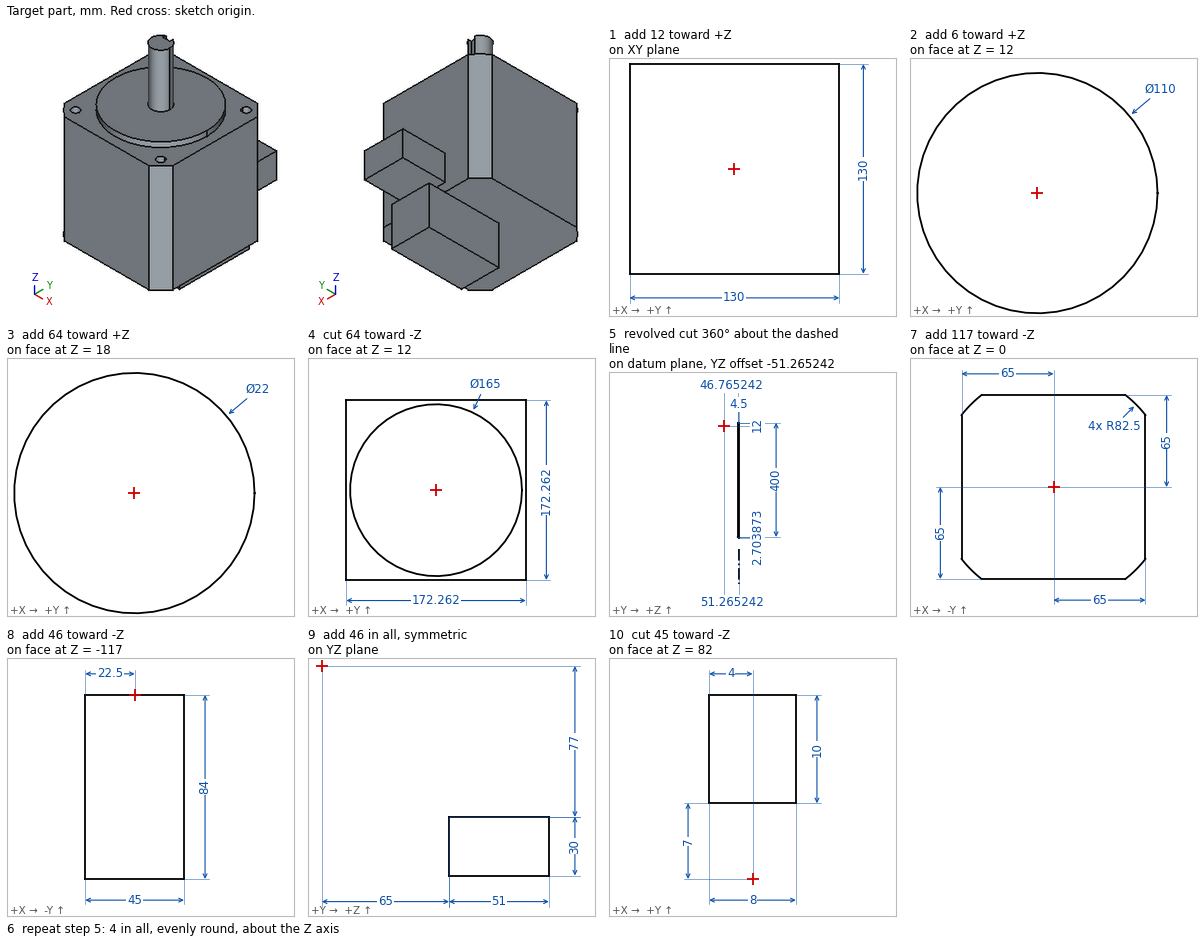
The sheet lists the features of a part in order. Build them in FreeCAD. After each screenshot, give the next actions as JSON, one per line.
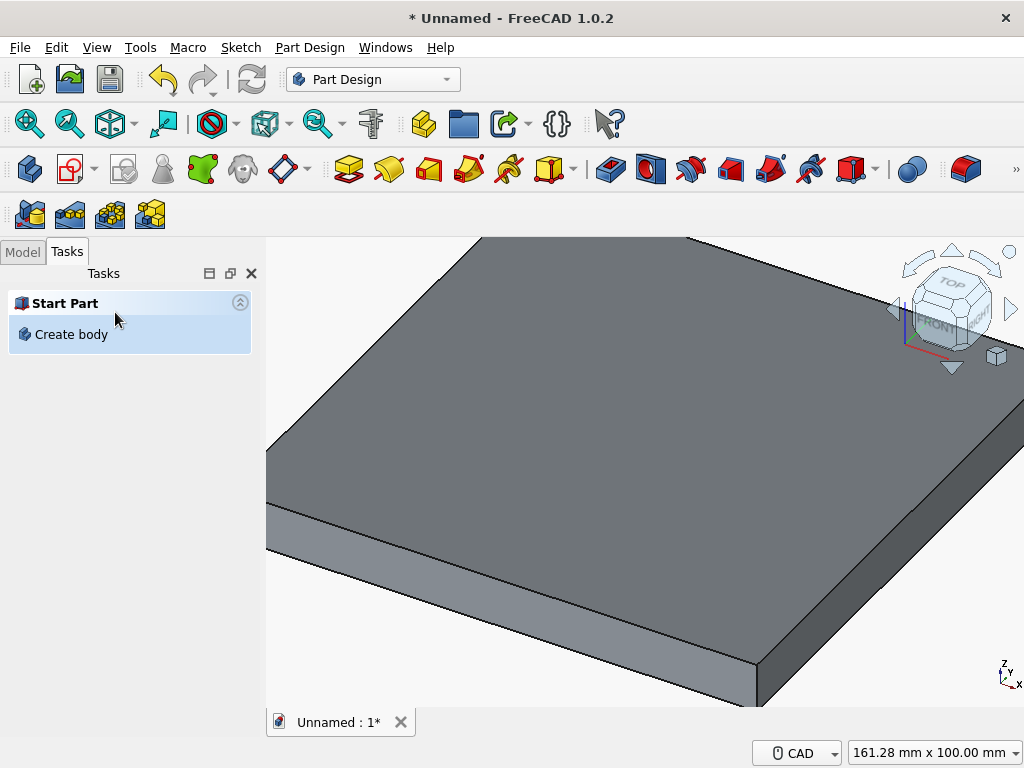
{"action": "left_click", "coordinate": [30, 124]}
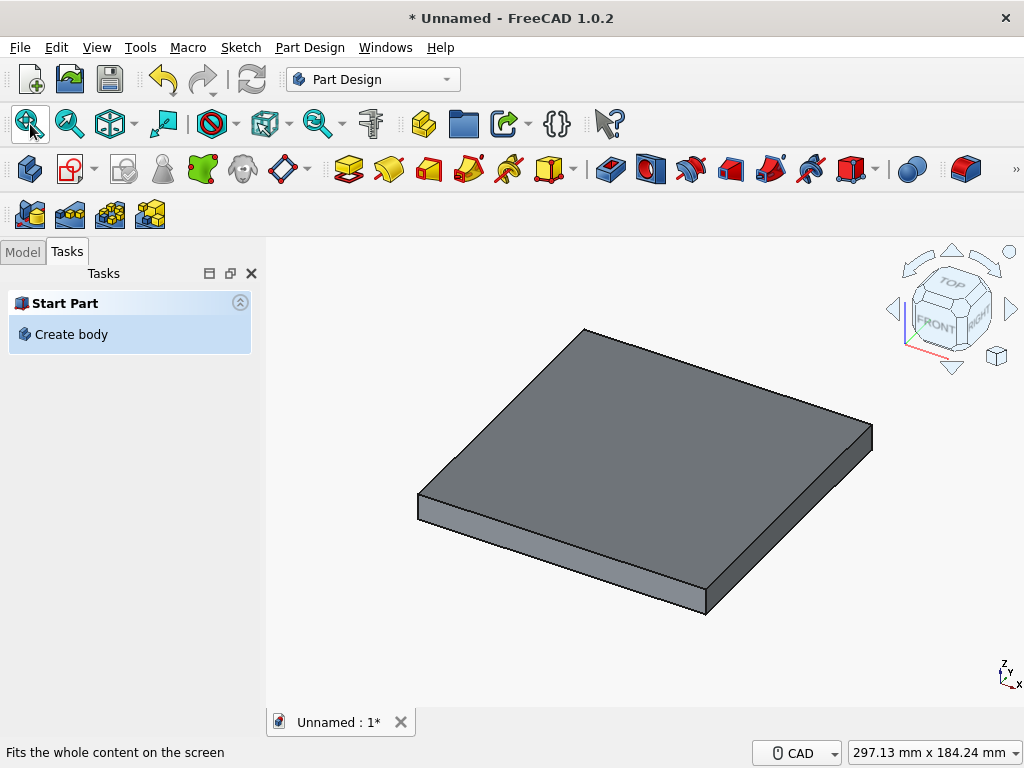
{"action": "left_click", "coordinate": [645, 458]}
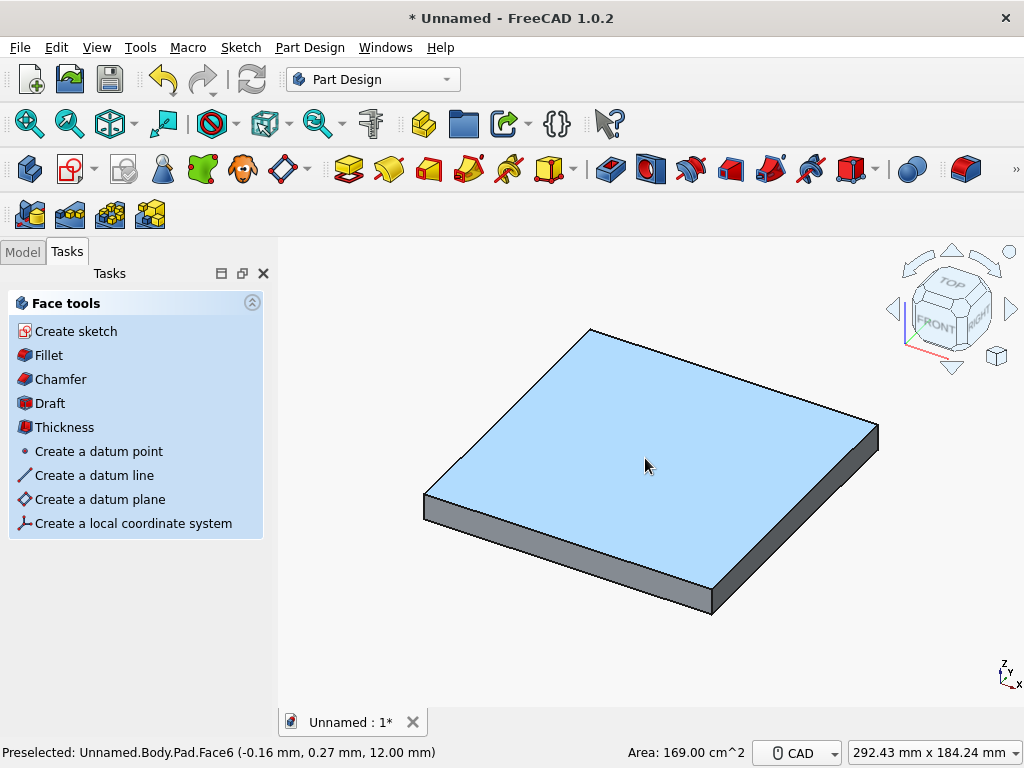
{"action": "left_click", "coordinate": [70, 170]}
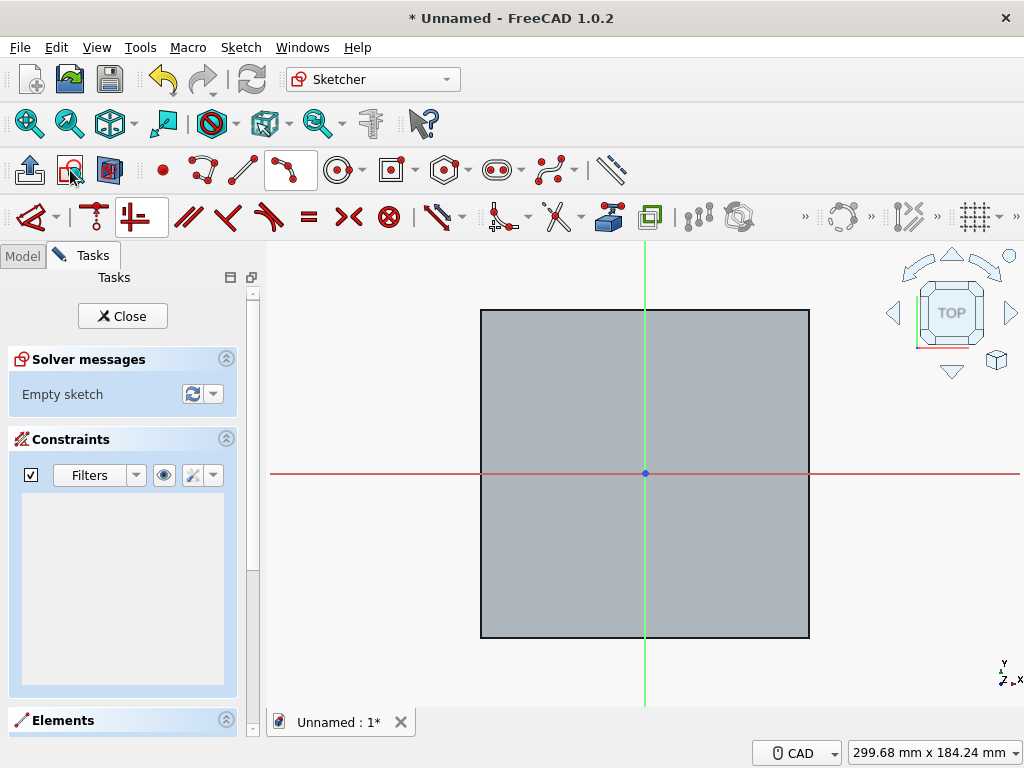
{"action": "left_click", "coordinate": [338, 170]}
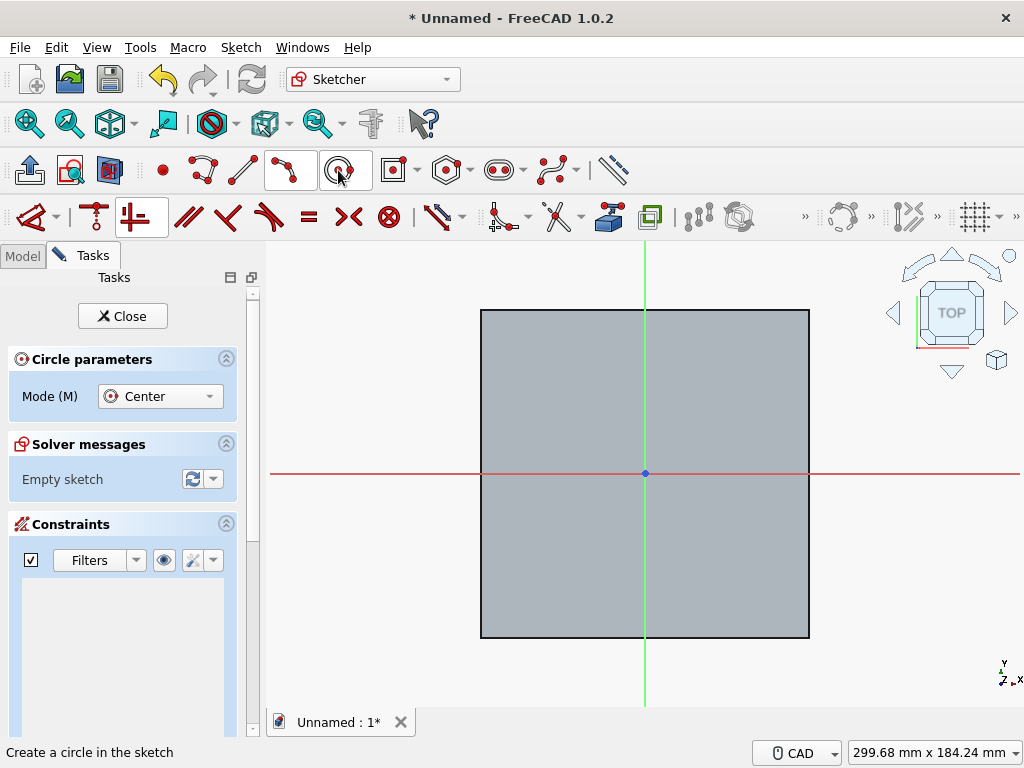
{"action": "left_click", "coordinate": [645, 474]}
{"action": "mouse_move", "coordinate": [743, 376]}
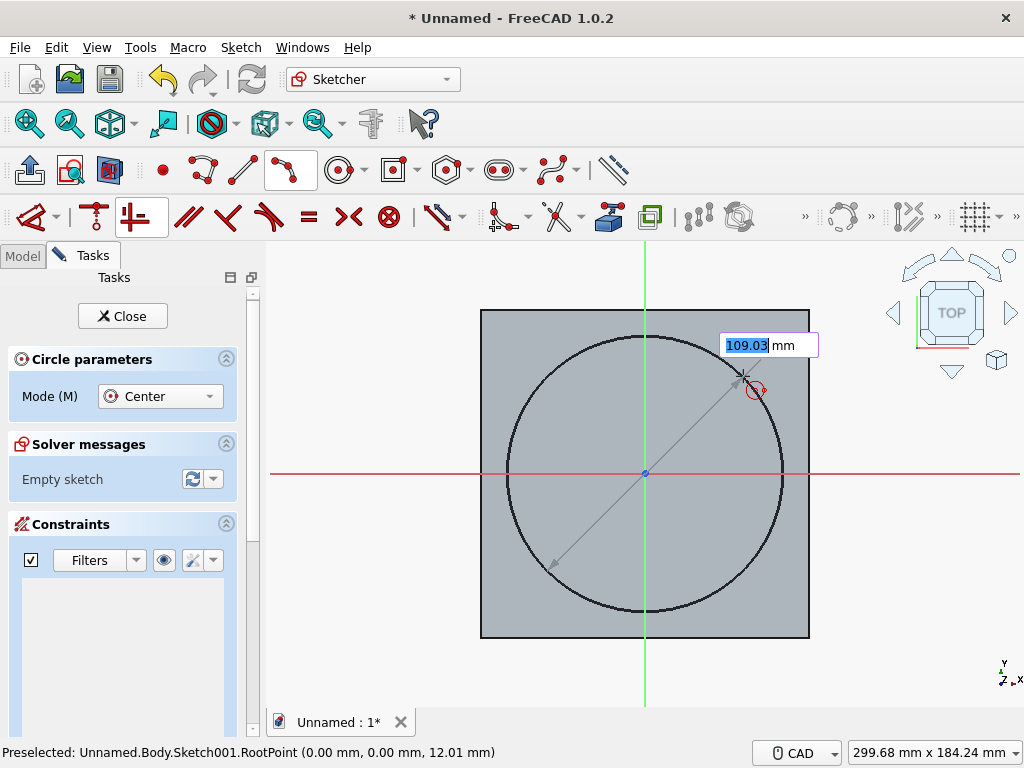
{"action": "type", "text": "110"}
{"action": "key", "text": "Return"}
{"action": "key", "text": "Escape"}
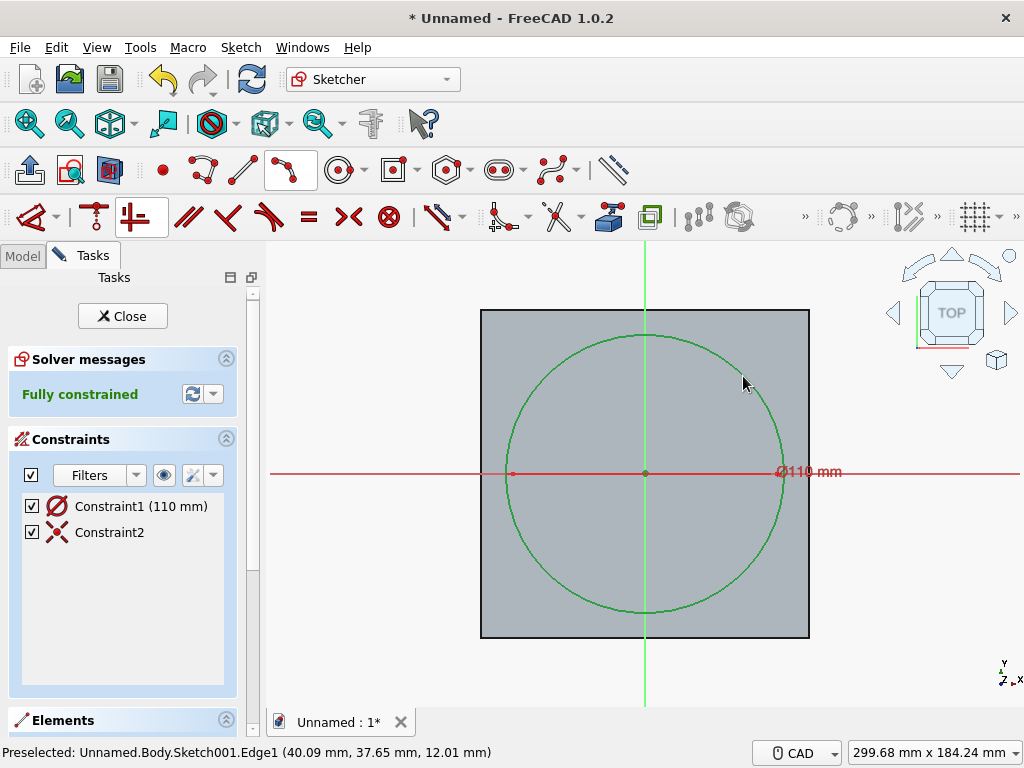
{"action": "left_click", "coordinate": [123, 316]}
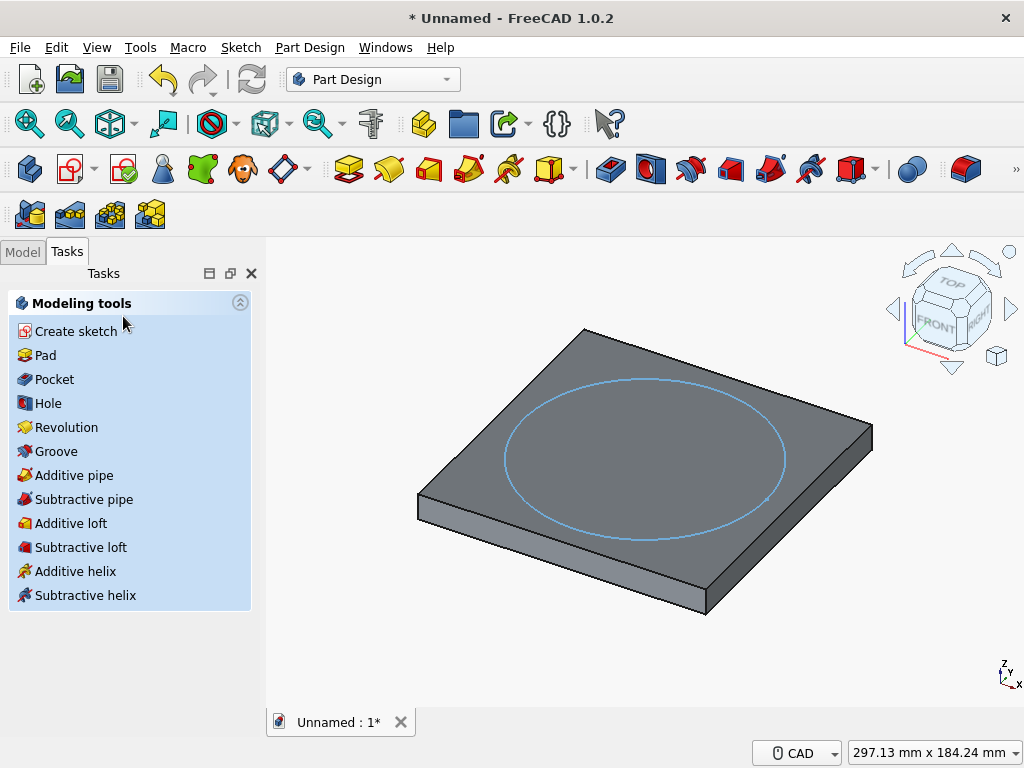
{"action": "left_click", "coordinate": [350, 170]}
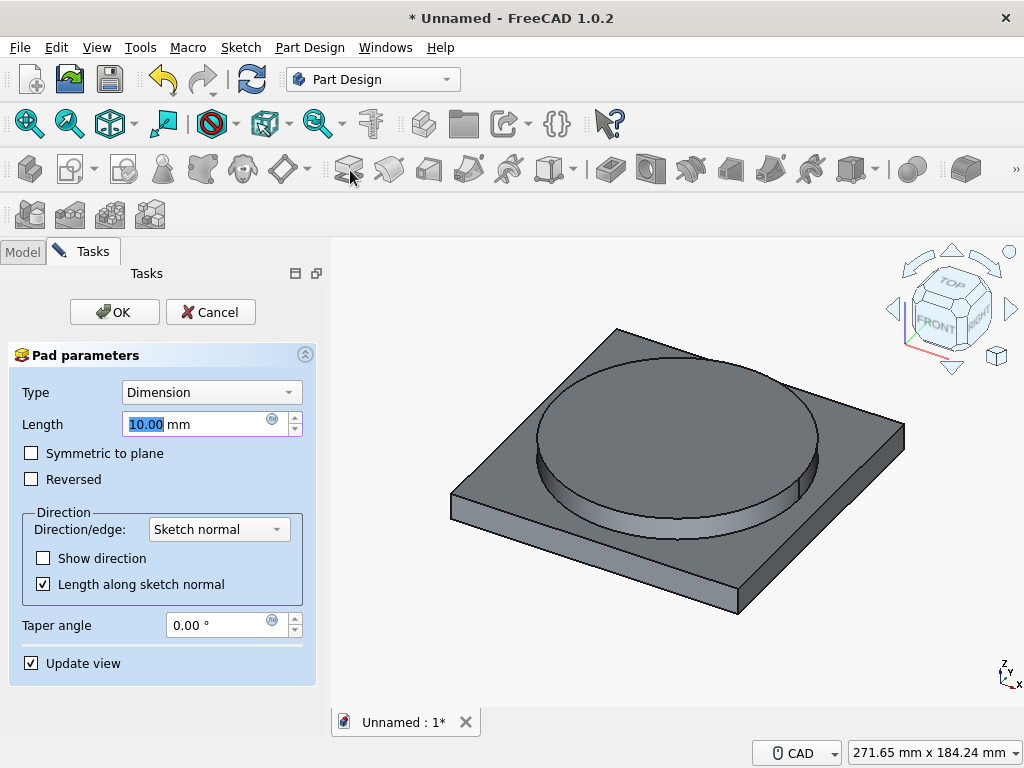
{"action": "type", "text": "6"}
{"action": "key", "text": "Tab"}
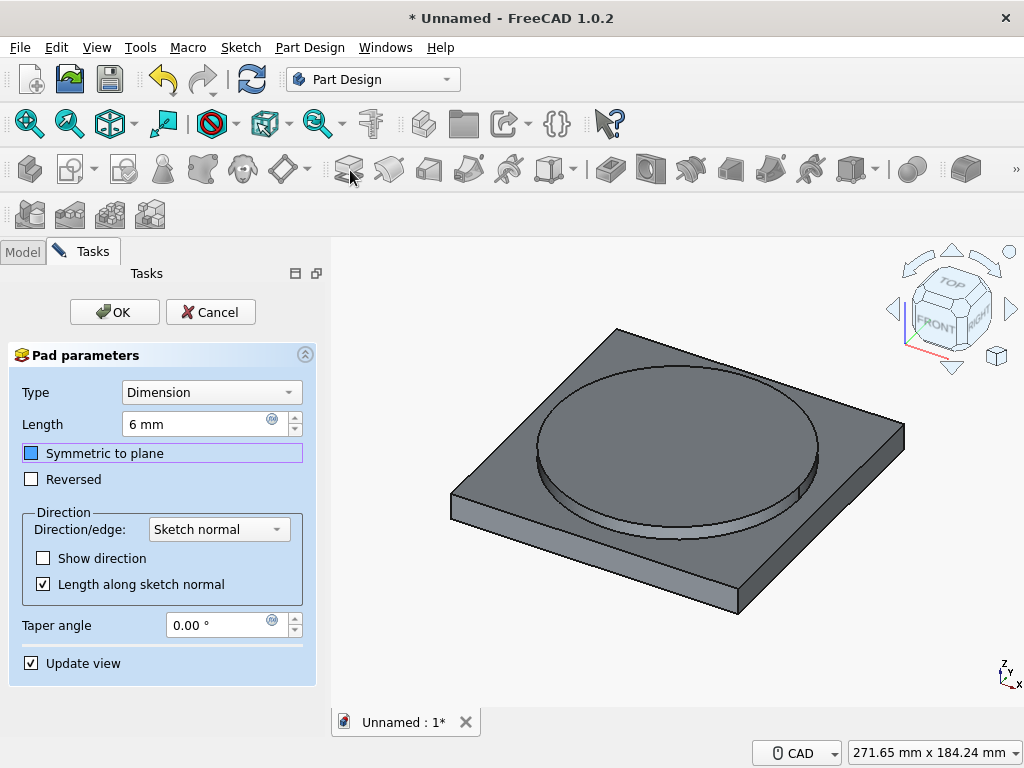
{"action": "left_click", "coordinate": [115, 312]}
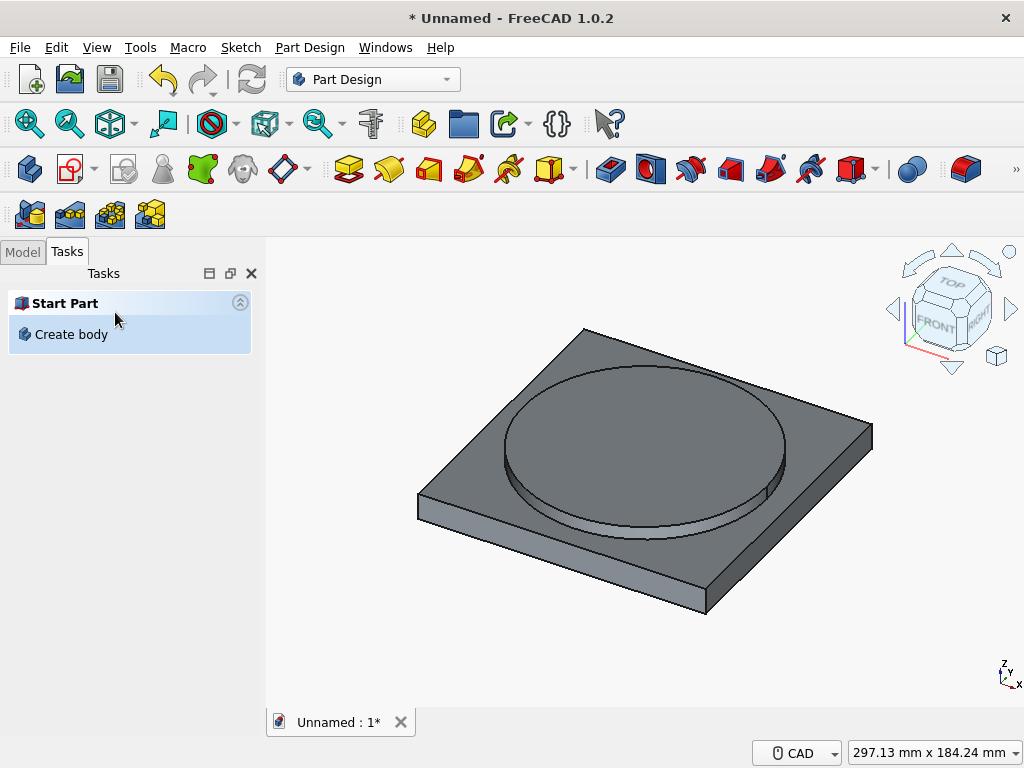
{"action": "left_click", "coordinate": [645, 446]}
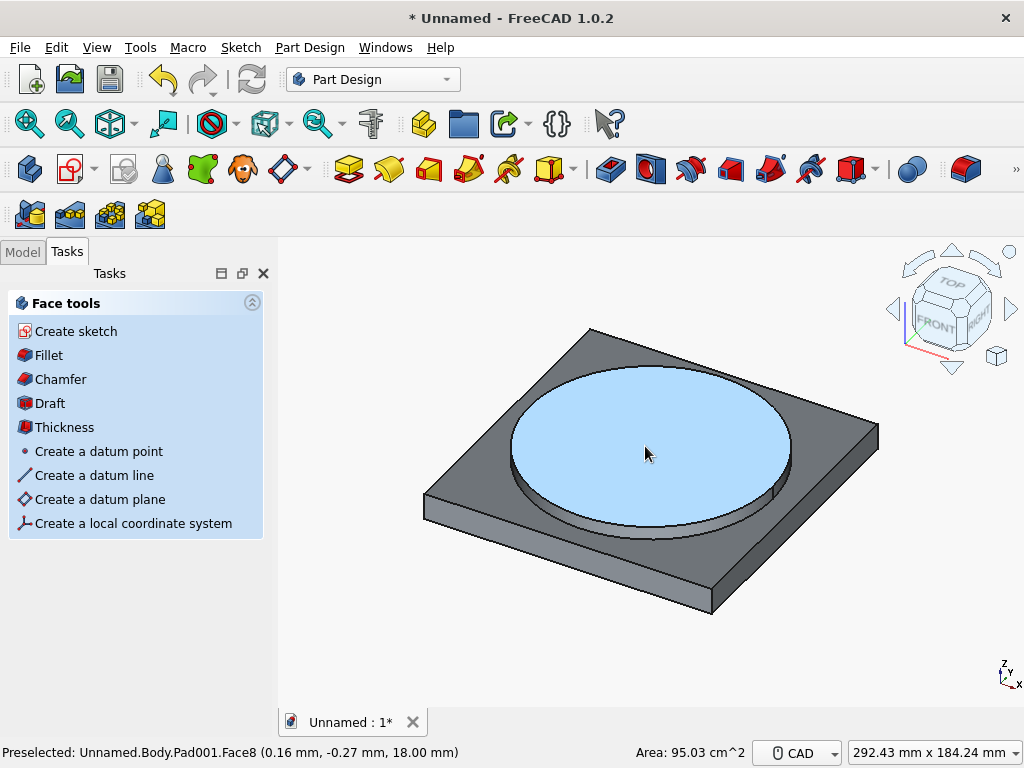
{"action": "left_click", "coordinate": [70, 170]}